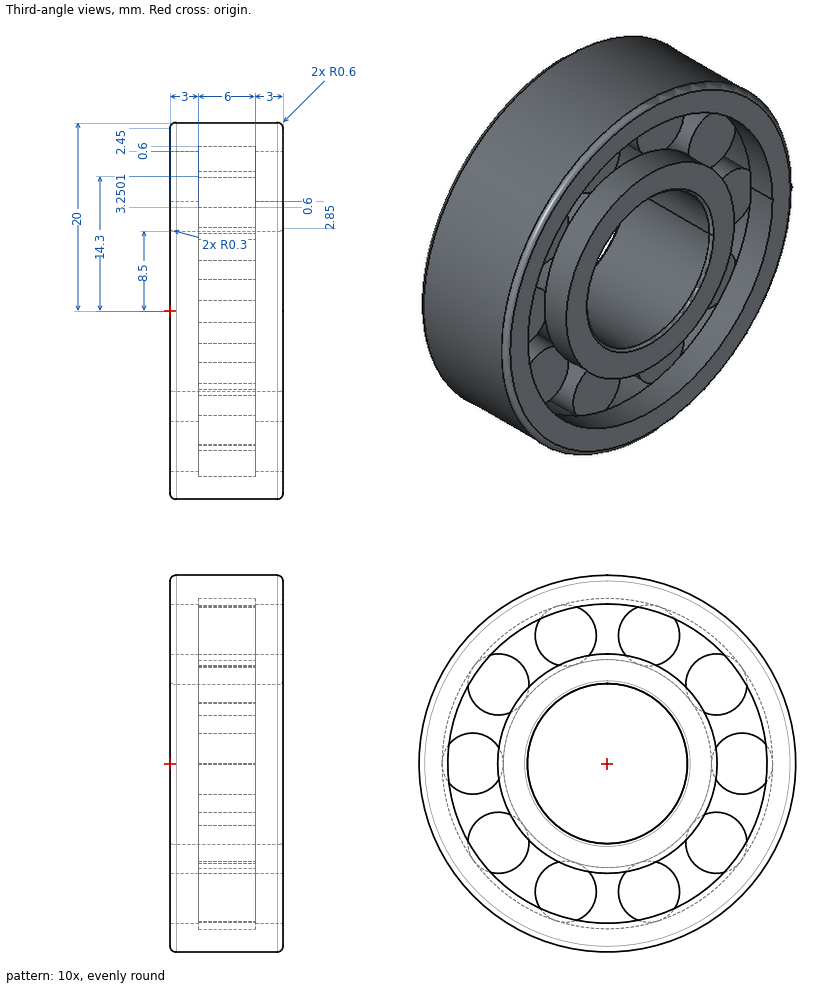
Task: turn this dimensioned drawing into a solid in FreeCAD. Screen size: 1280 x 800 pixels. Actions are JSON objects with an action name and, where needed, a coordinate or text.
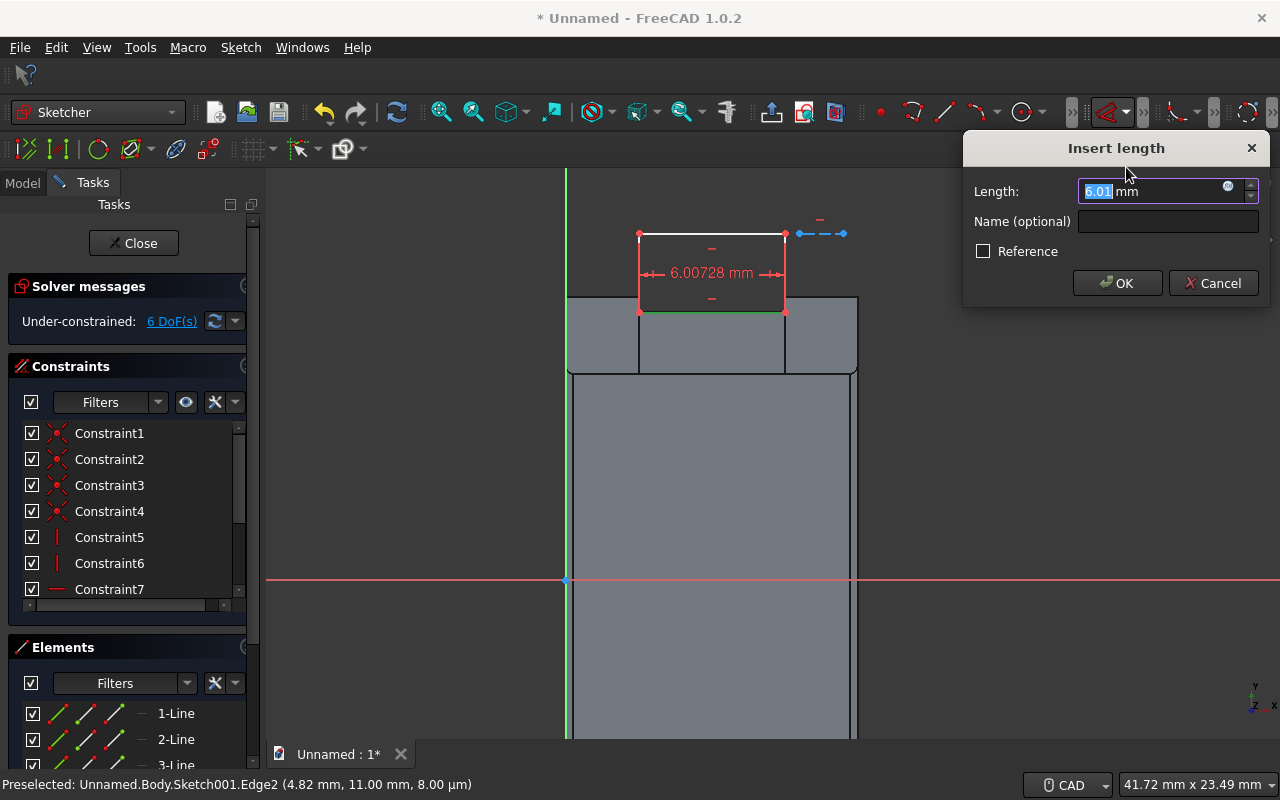
{"action": "type", "text": "6"}
{"action": "key", "text": "Return"}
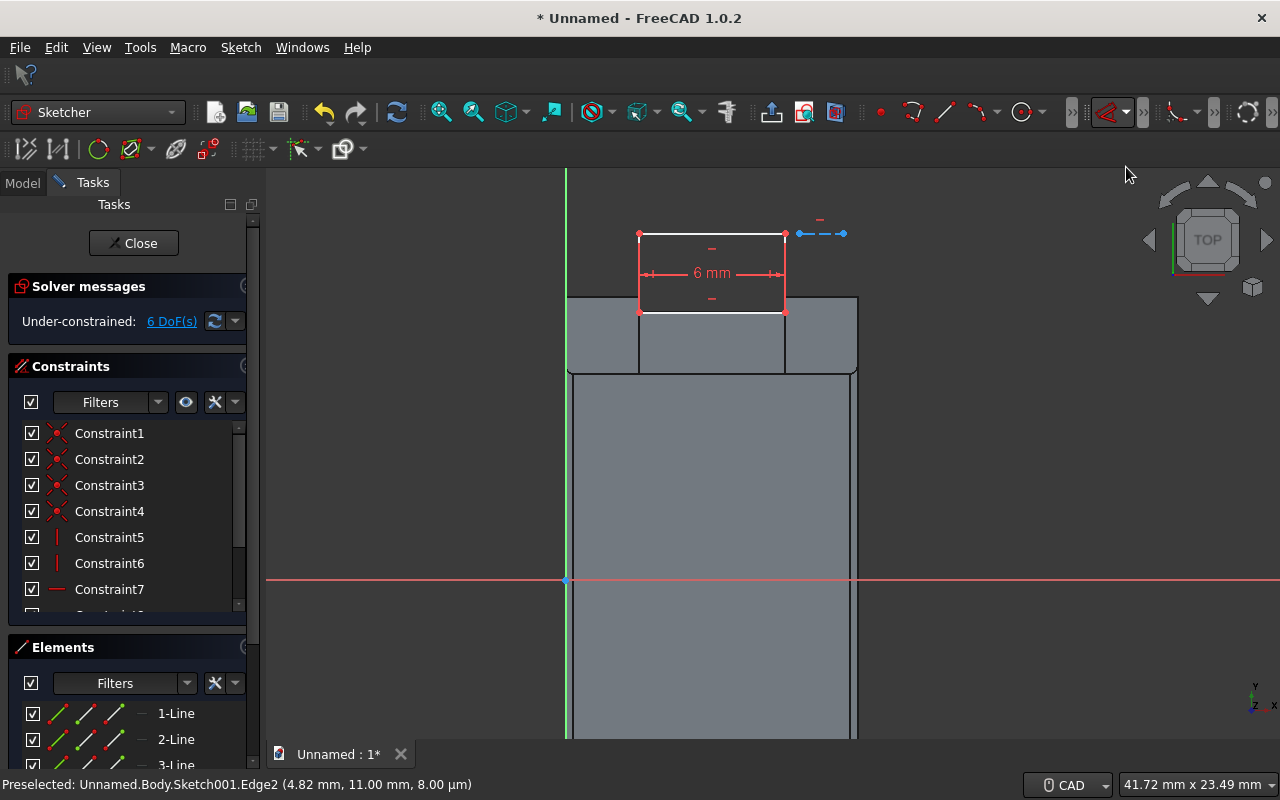
{"action": "left_click", "coordinate": [639, 234]}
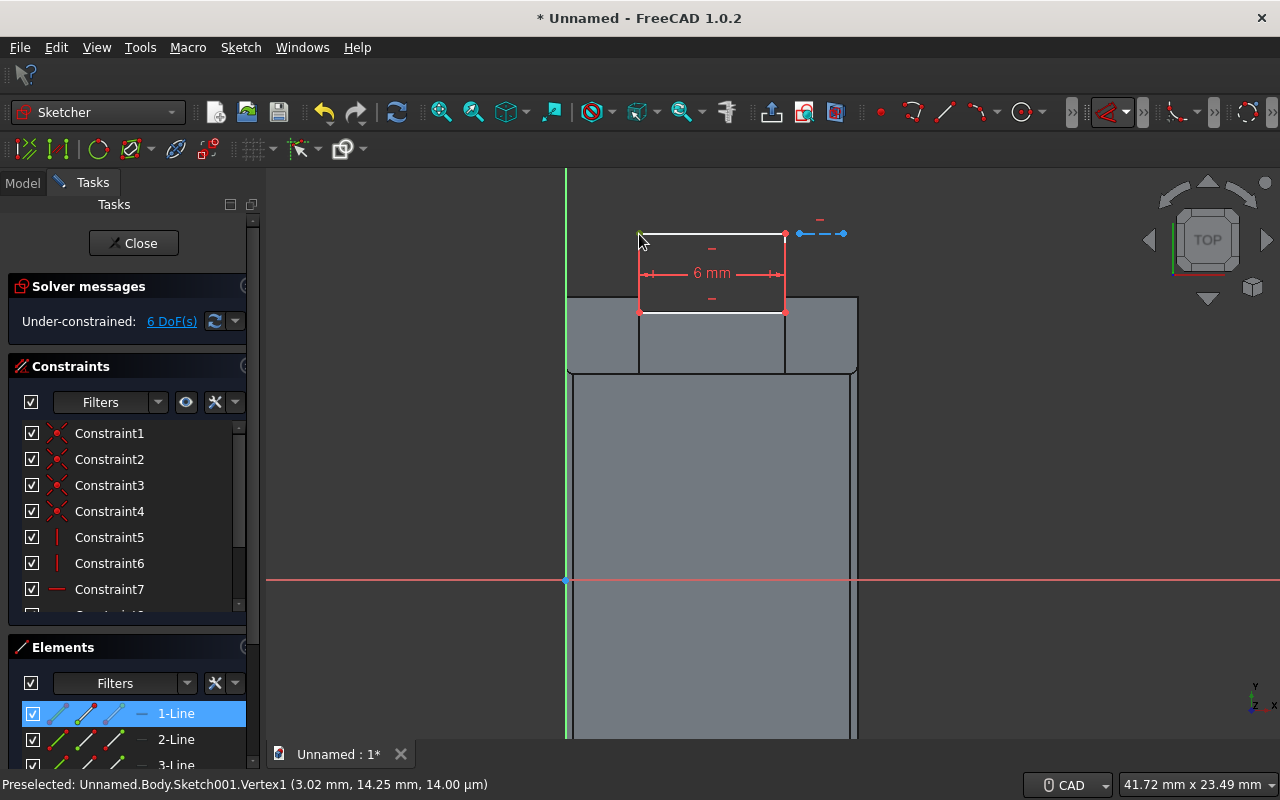
{"action": "left_click", "coordinate": [1128, 112]}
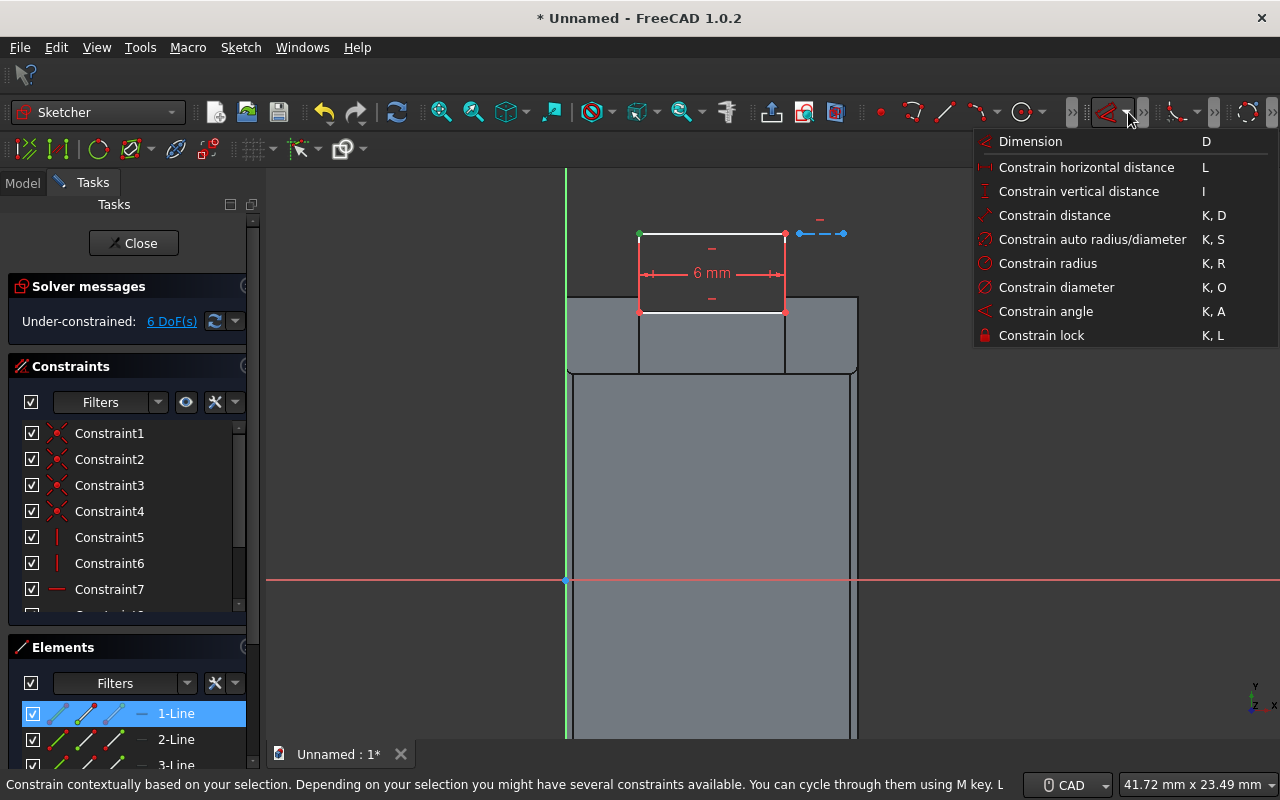
{"action": "left_click", "coordinate": [1126, 167]}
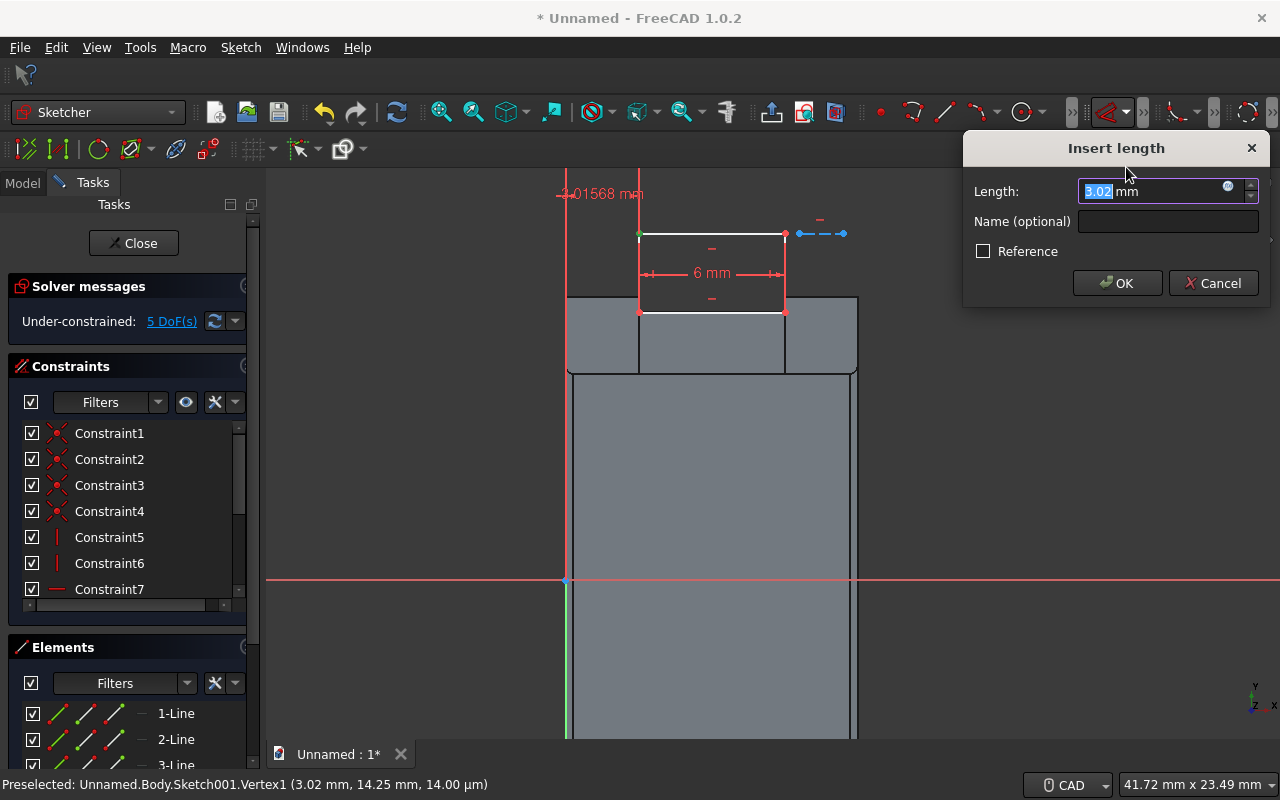
{"action": "type", "text": "3"}
{"action": "key", "text": "Return"}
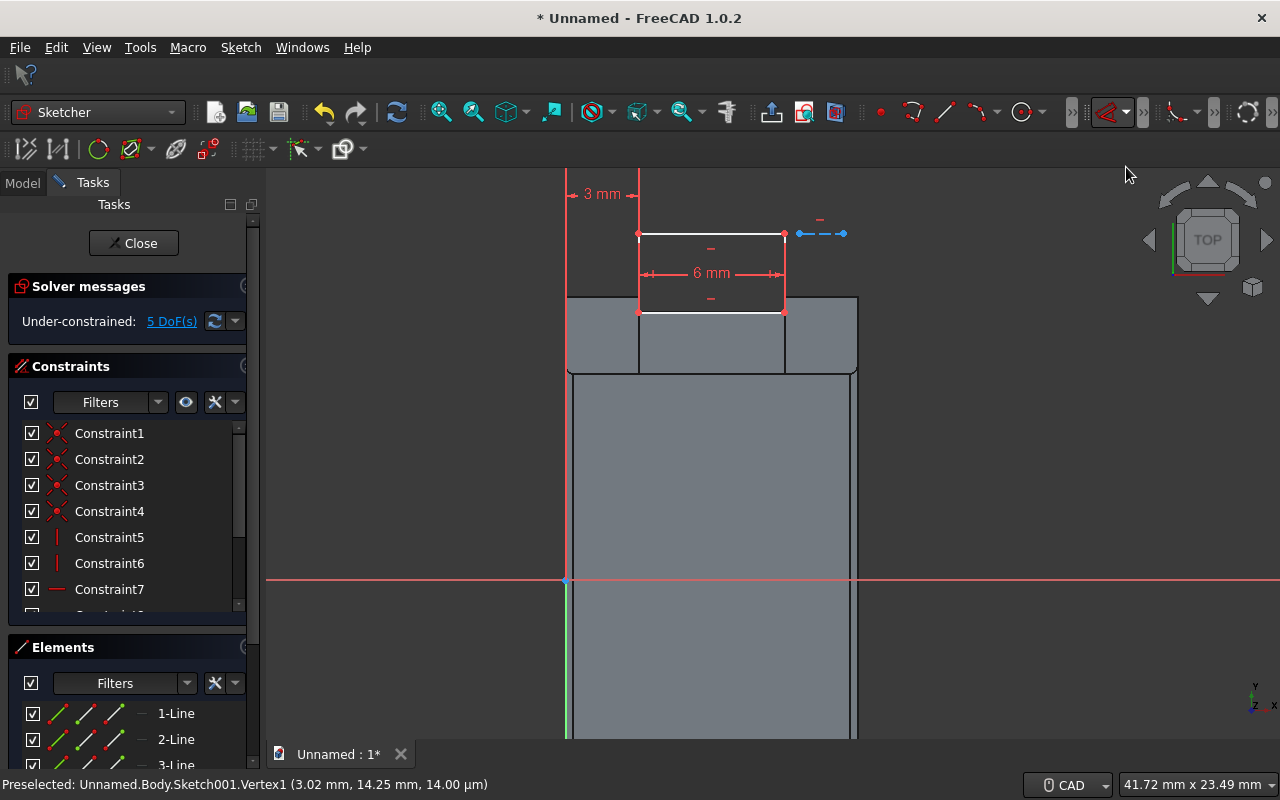
{"action": "left_click", "coordinate": [639, 234]}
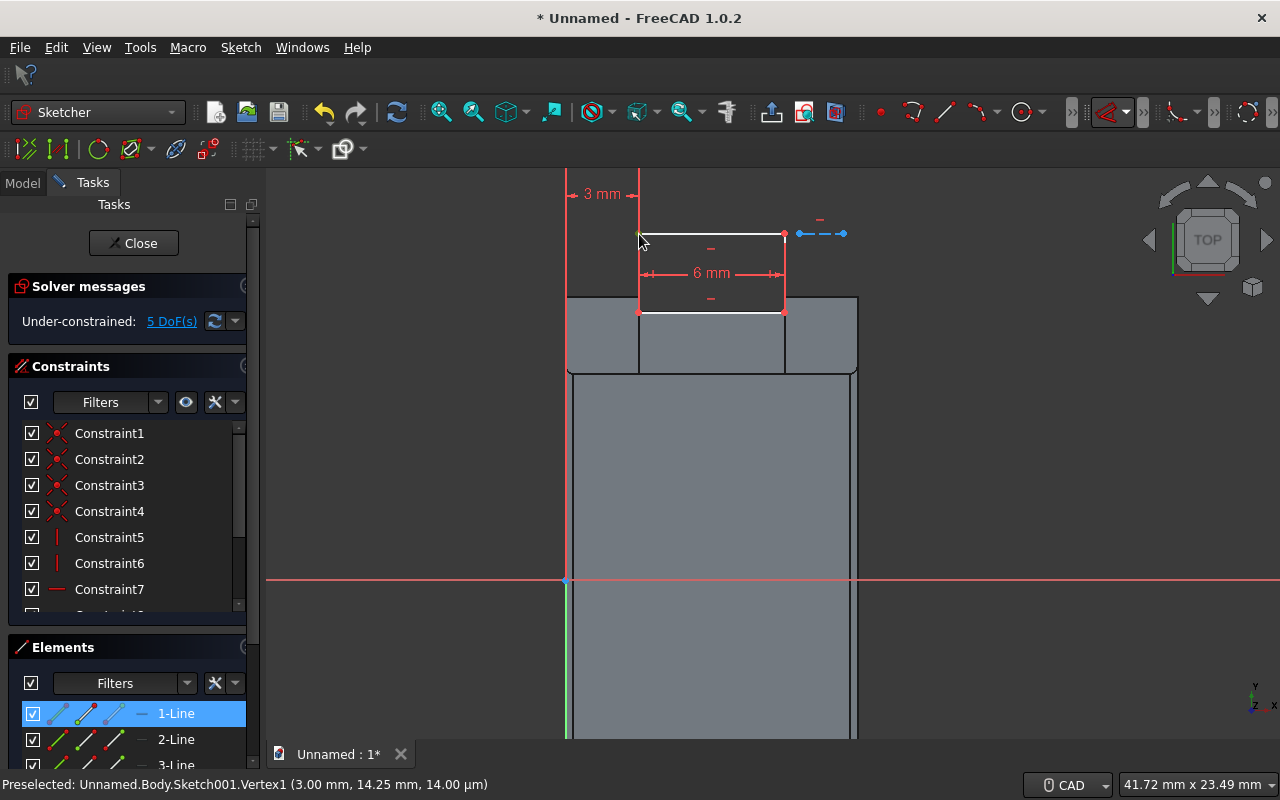
{"action": "key", "text": "i"}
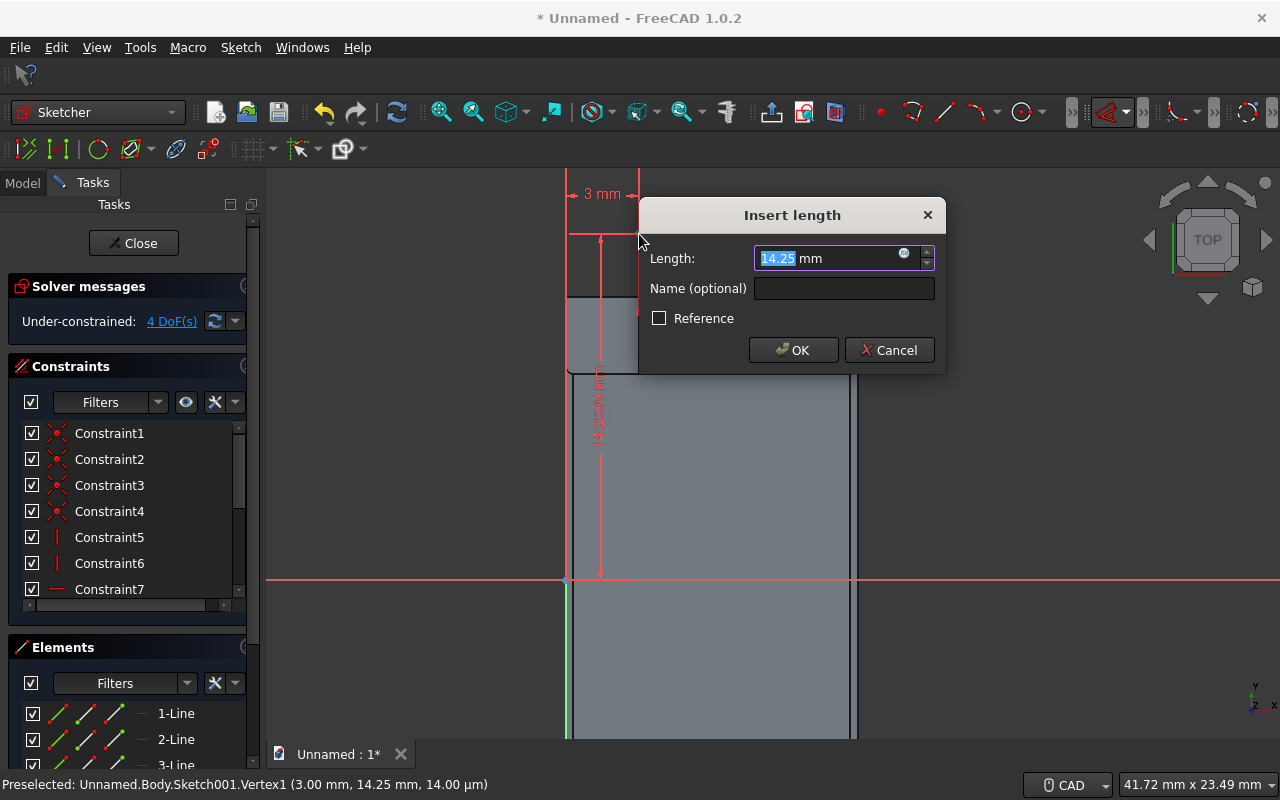
{"action": "type", "text": "14.3"}
{"action": "key", "text": "Return"}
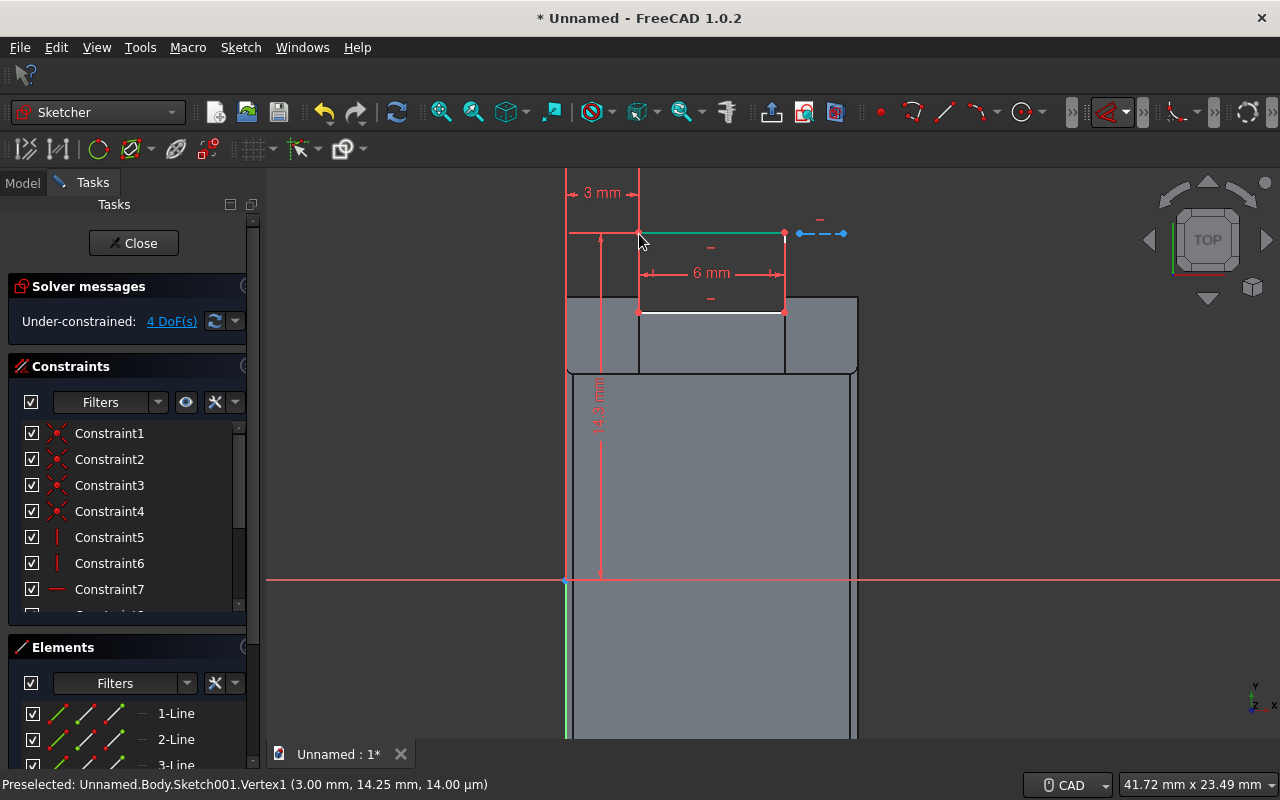
{"action": "left_click", "coordinate": [799, 234]}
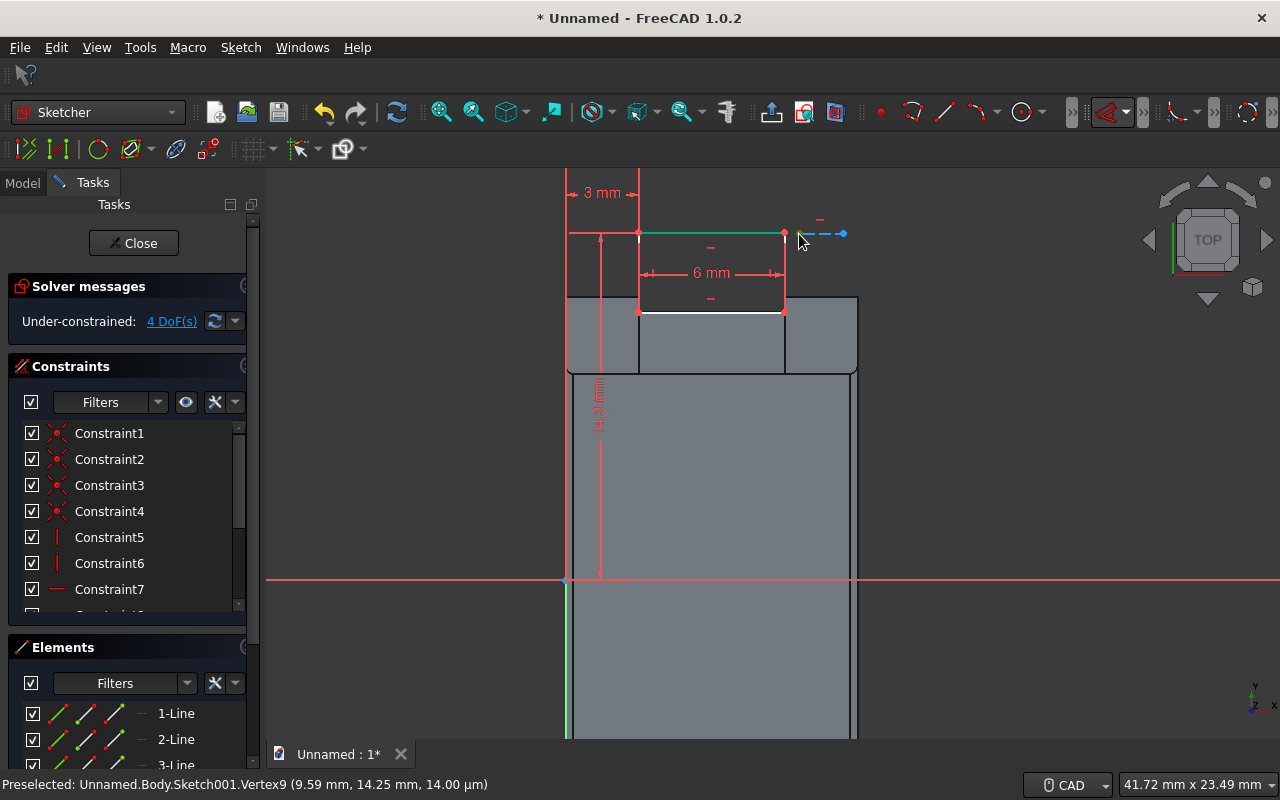
{"action": "key", "text": "i"}